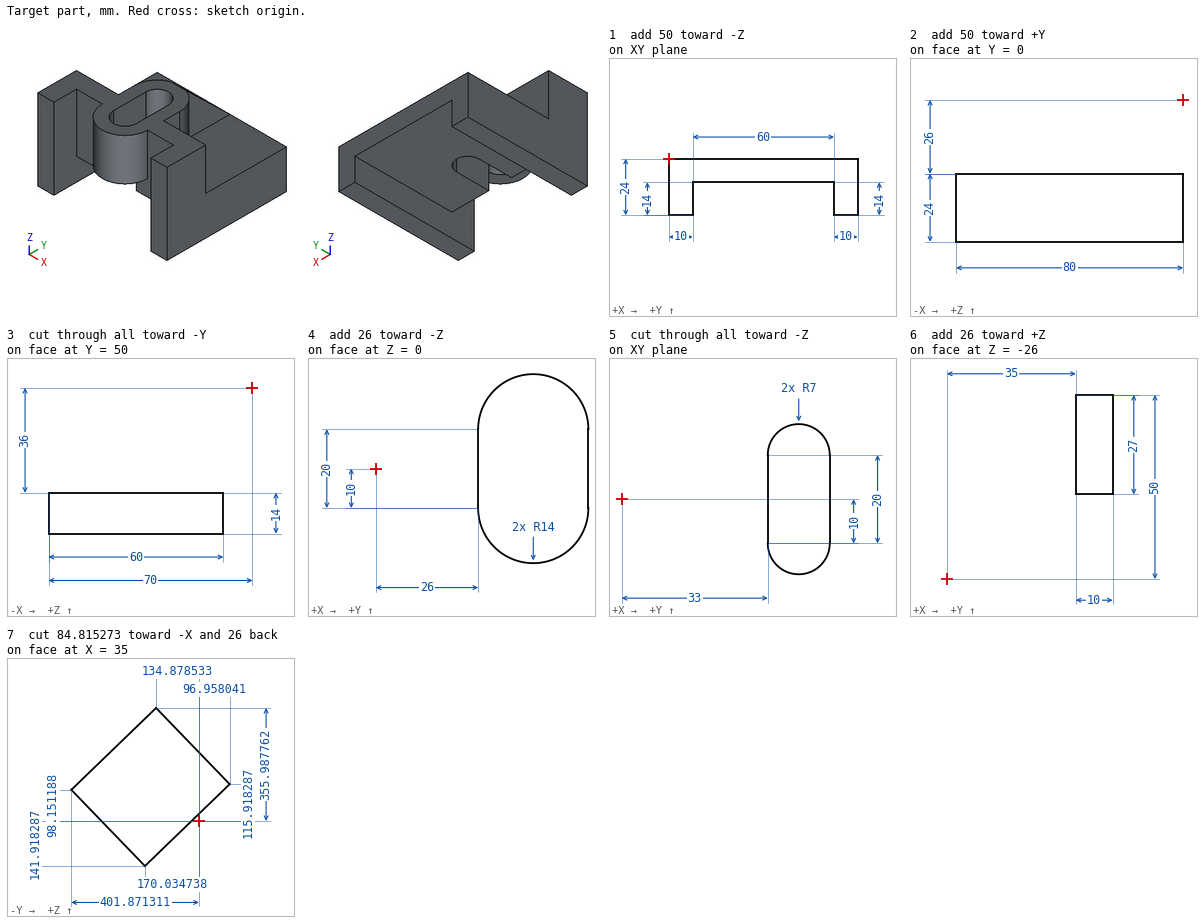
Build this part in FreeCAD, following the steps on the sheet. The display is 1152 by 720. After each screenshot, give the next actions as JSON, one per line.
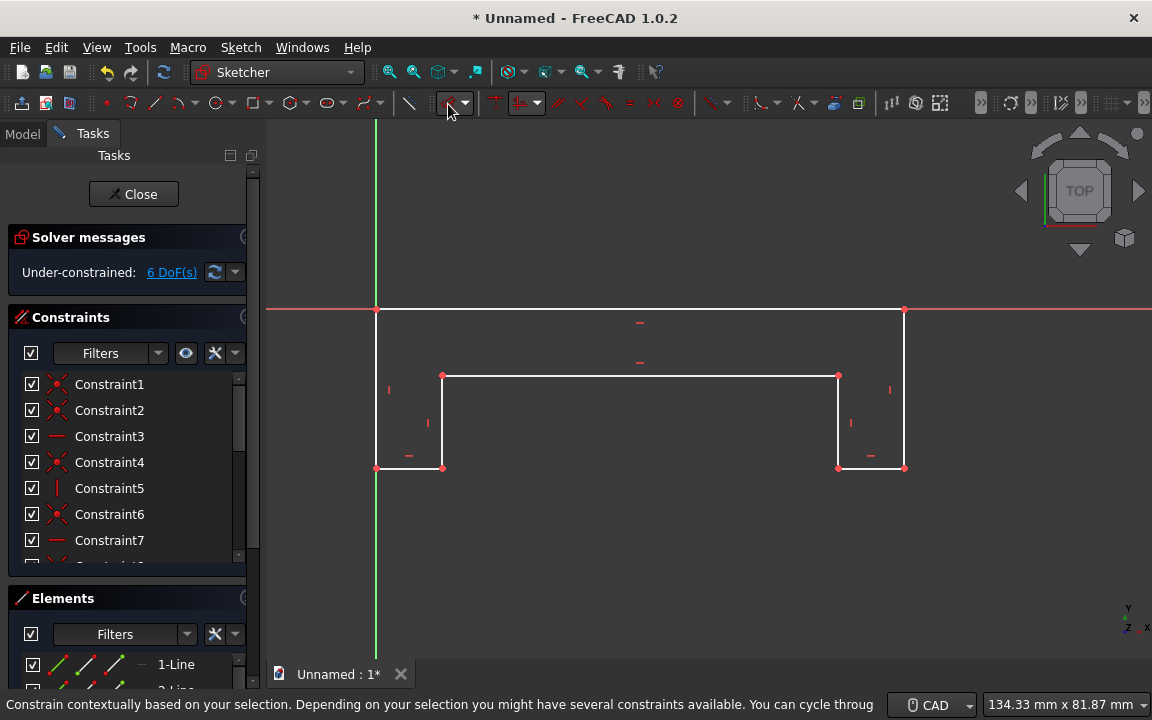
{"action": "left_click", "coordinate": [376, 357]}
{"action": "left_click", "coordinate": [342, 389]}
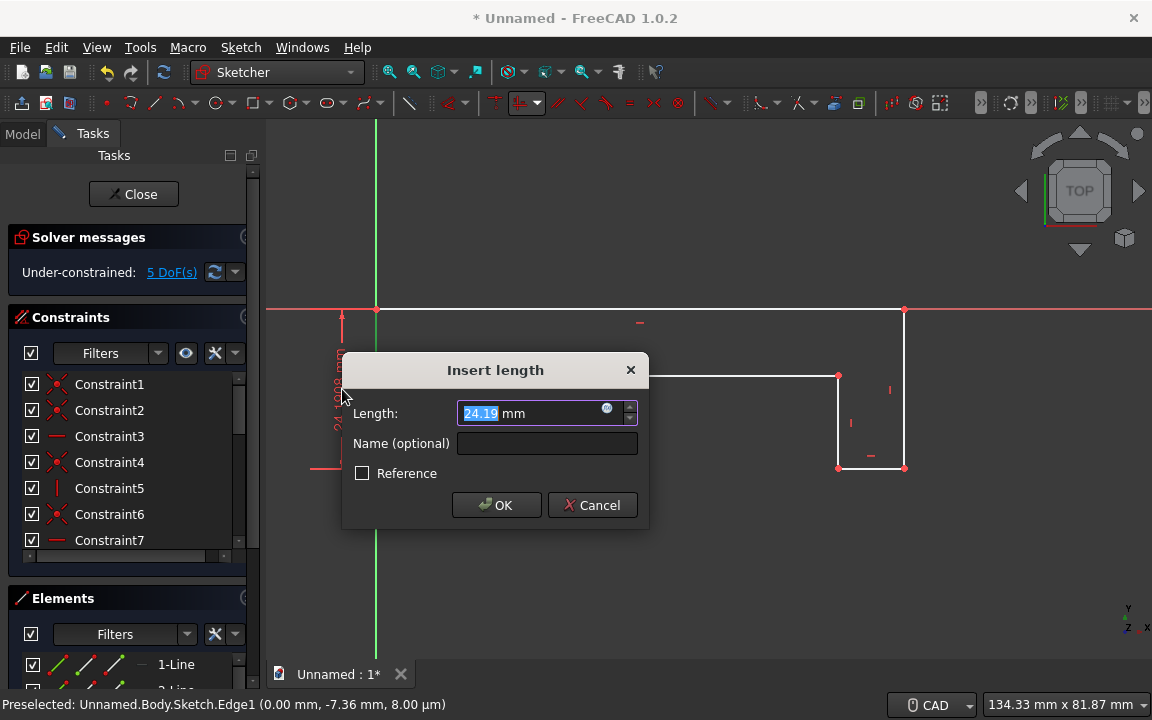
{"action": "type", "text": "24"}
{"action": "key", "text": "Return"}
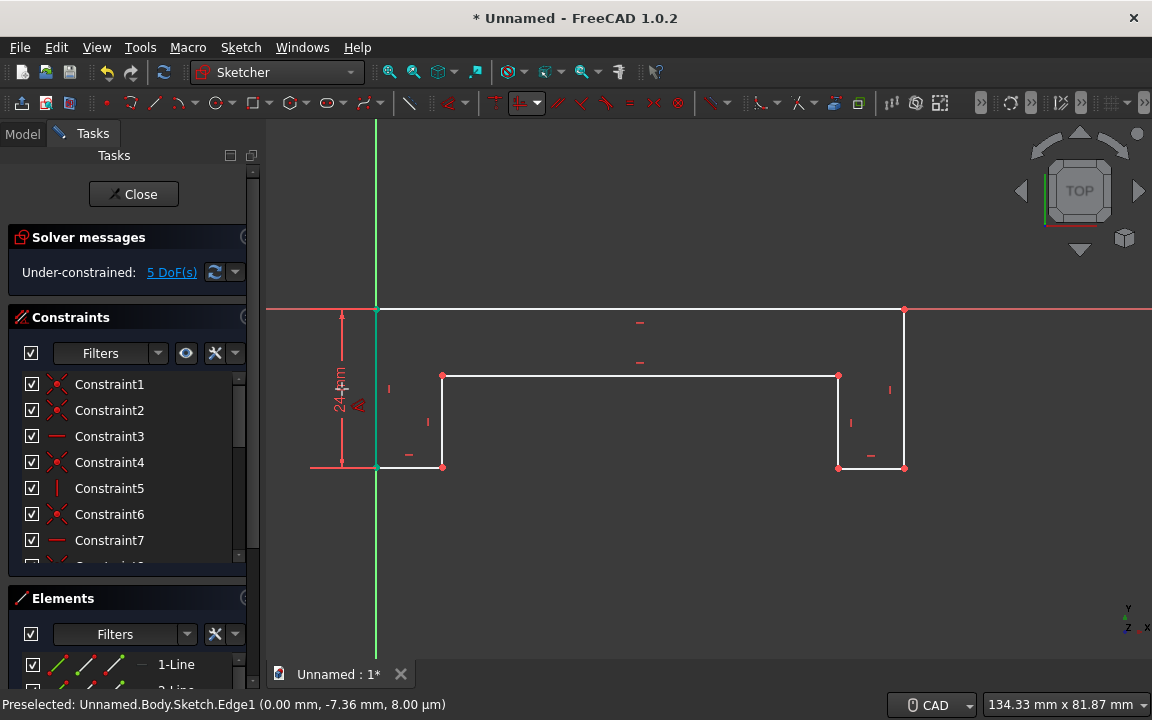
{"action": "left_click", "coordinate": [396, 468]}
{"action": "left_click", "coordinate": [409, 502]}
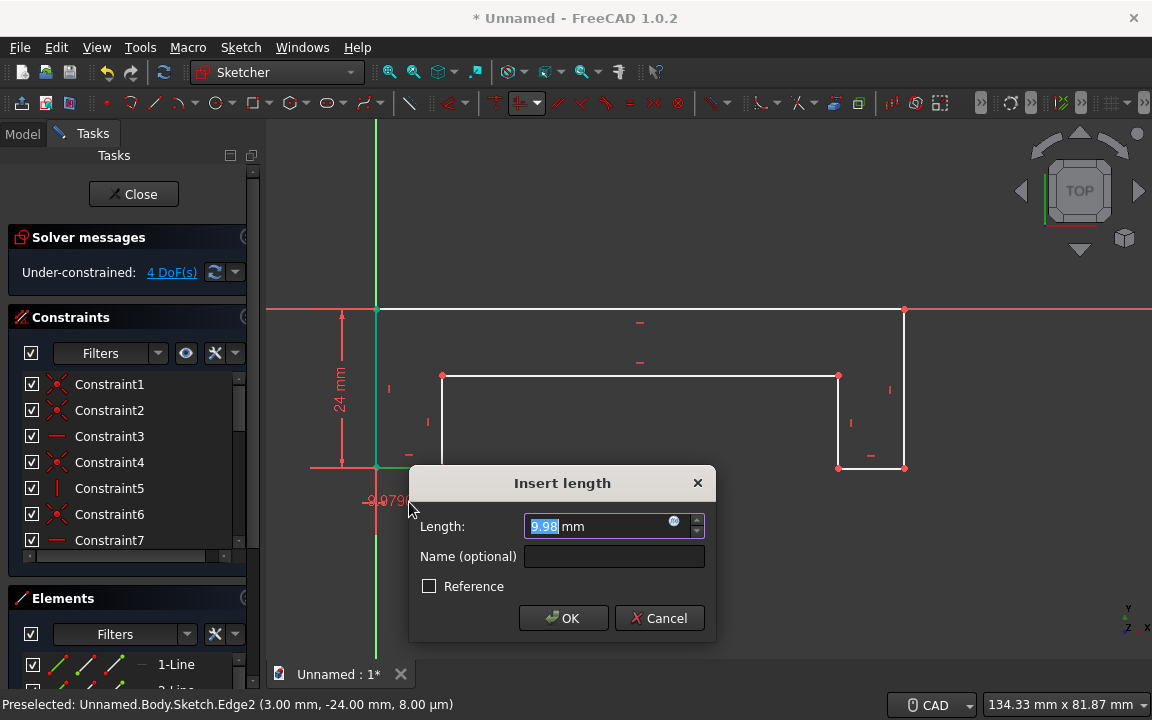
{"action": "type", "text": "10"}
{"action": "key", "text": "Return"}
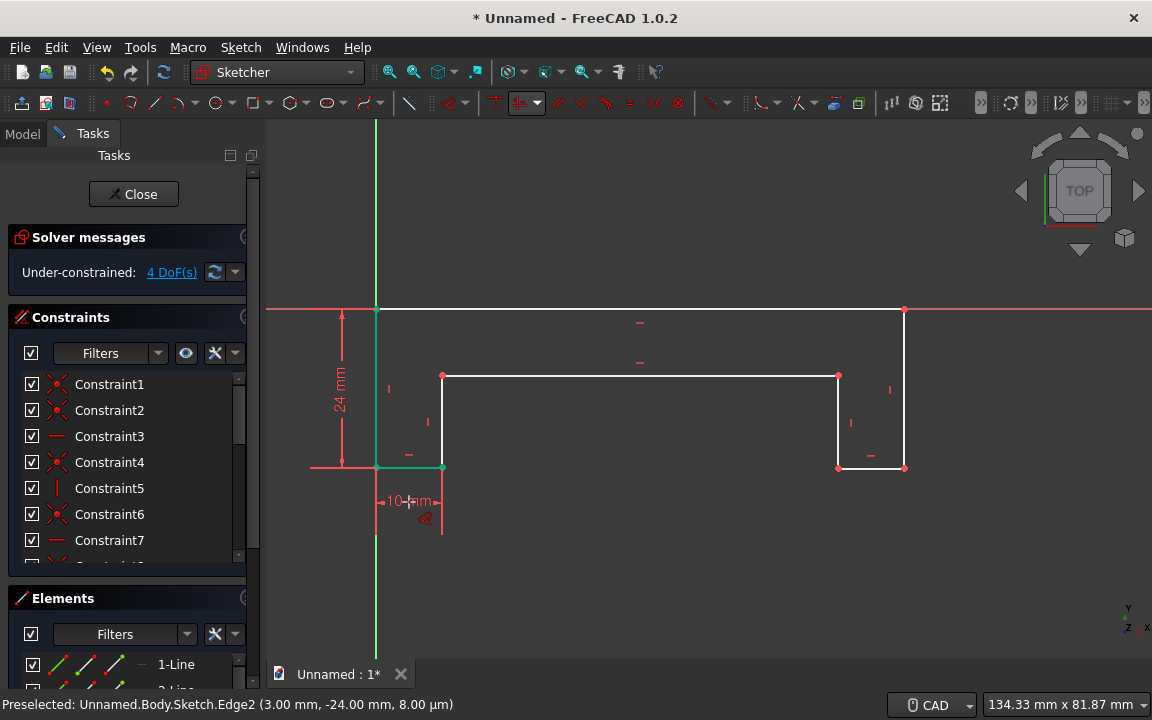
{"action": "left_click", "coordinate": [442, 440]}
{"action": "left_click", "coordinate": [408, 422]}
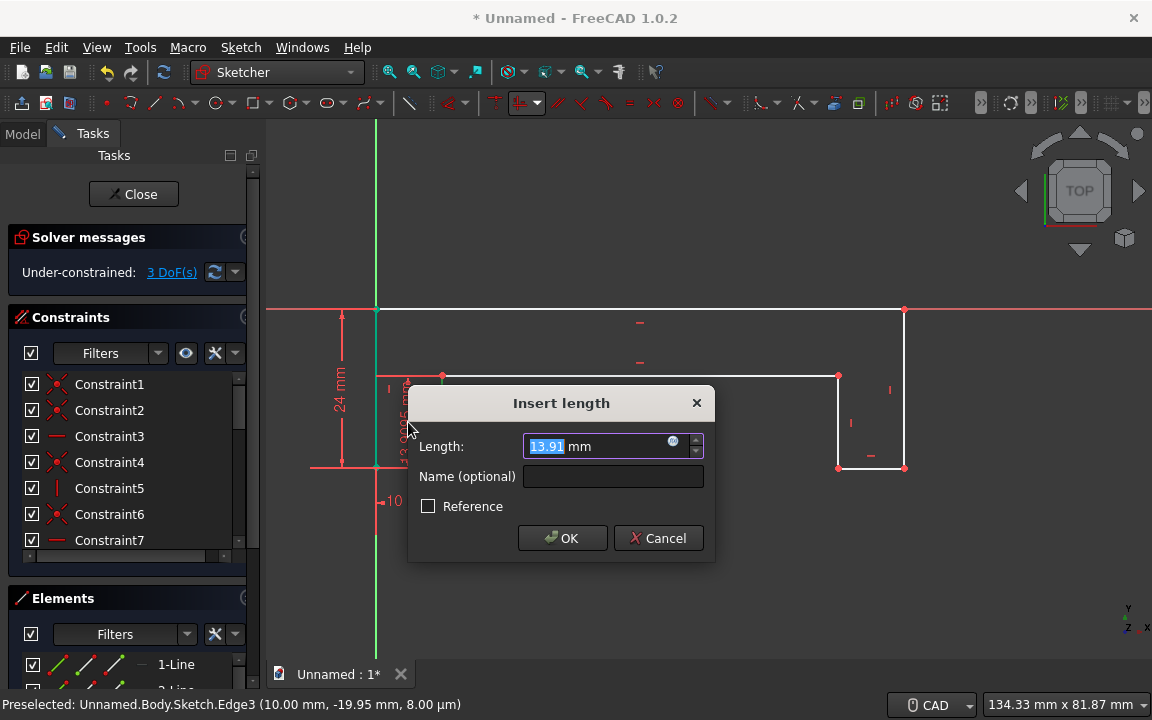
{"action": "type", "text": "14"}
{"action": "key", "text": "Return"}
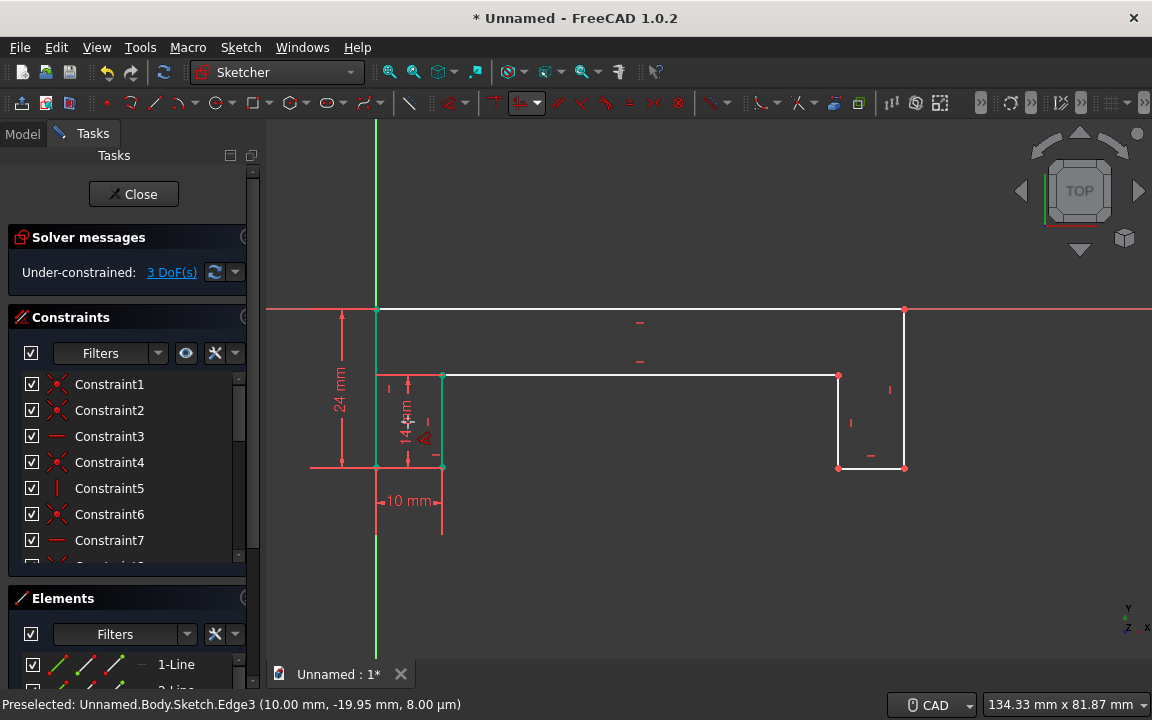
{"action": "left_click", "coordinate": [561, 375]}
{"action": "left_click", "coordinate": [640, 341]}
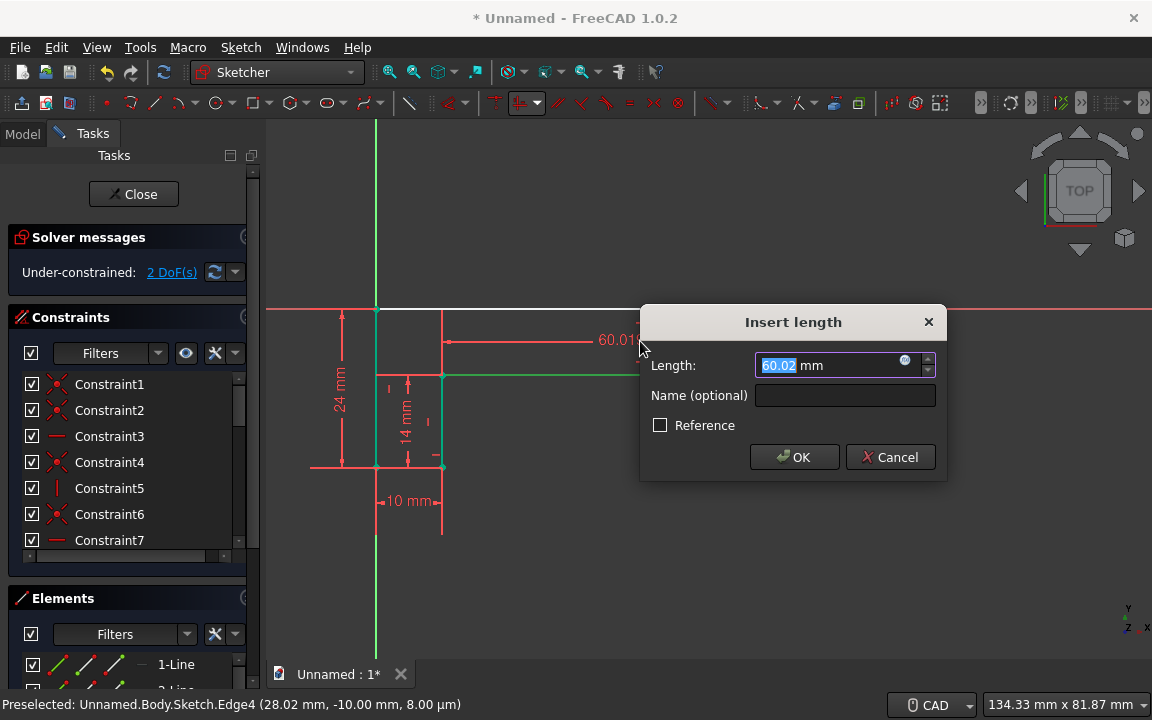
{"action": "type", "text": "60"}
{"action": "key", "text": "Return"}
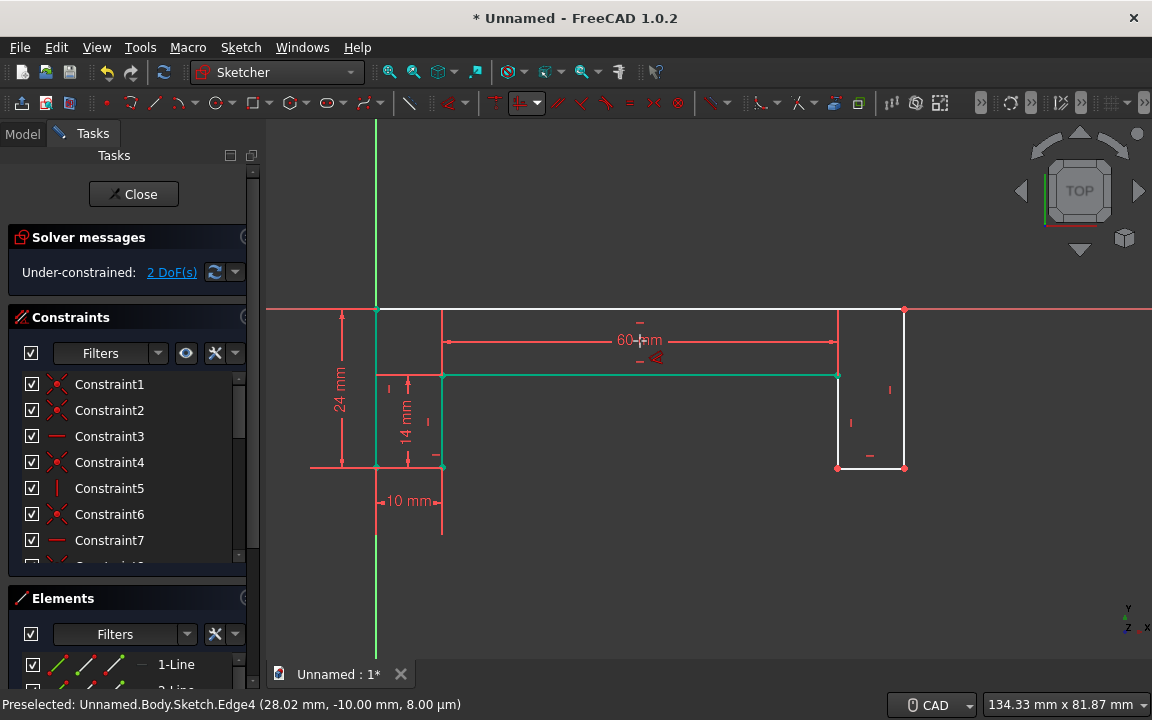
{"action": "left_click", "coordinate": [838, 403]}
{"action": "left_click", "coordinate": [872, 422]}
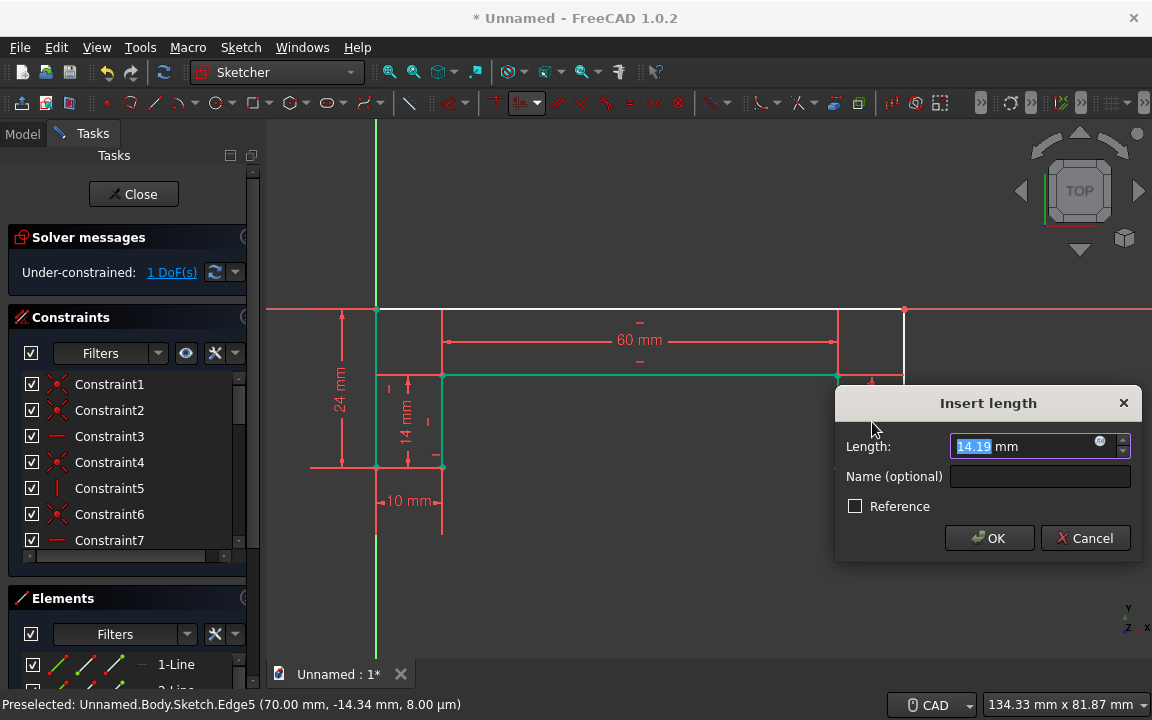
{"action": "type", "text": "14"}
{"action": "key", "text": "Return"}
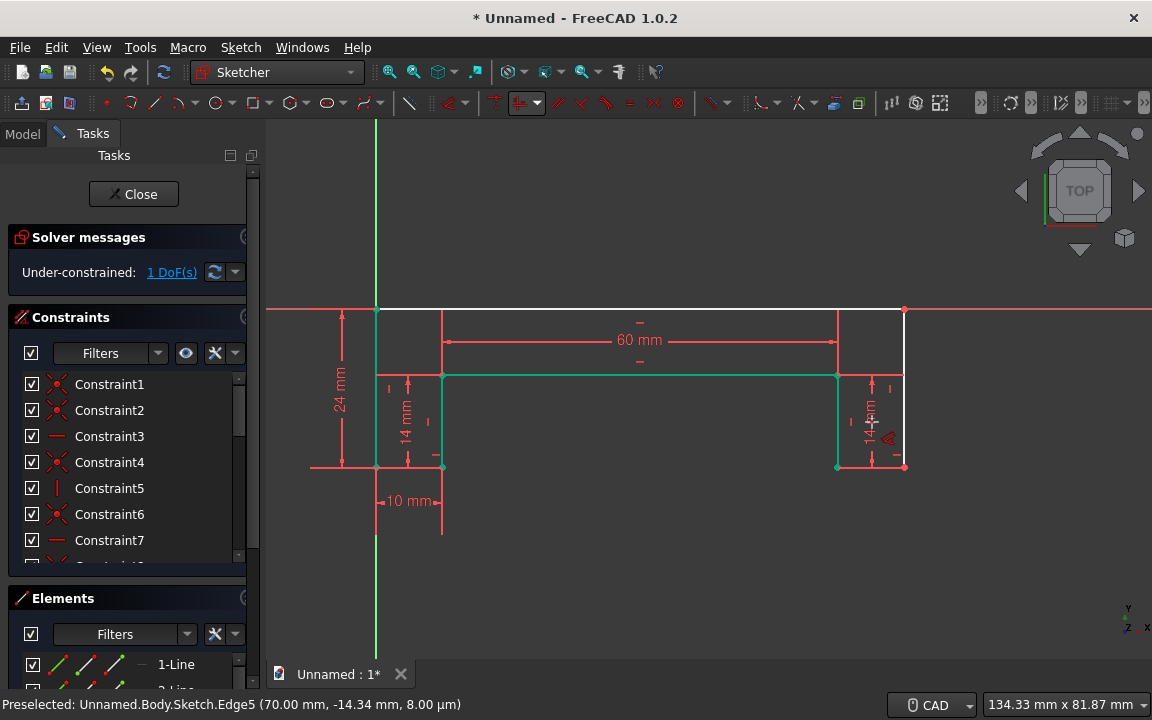
{"action": "left_click", "coordinate": [858, 468]}
{"action": "left_click", "coordinate": [871, 502]}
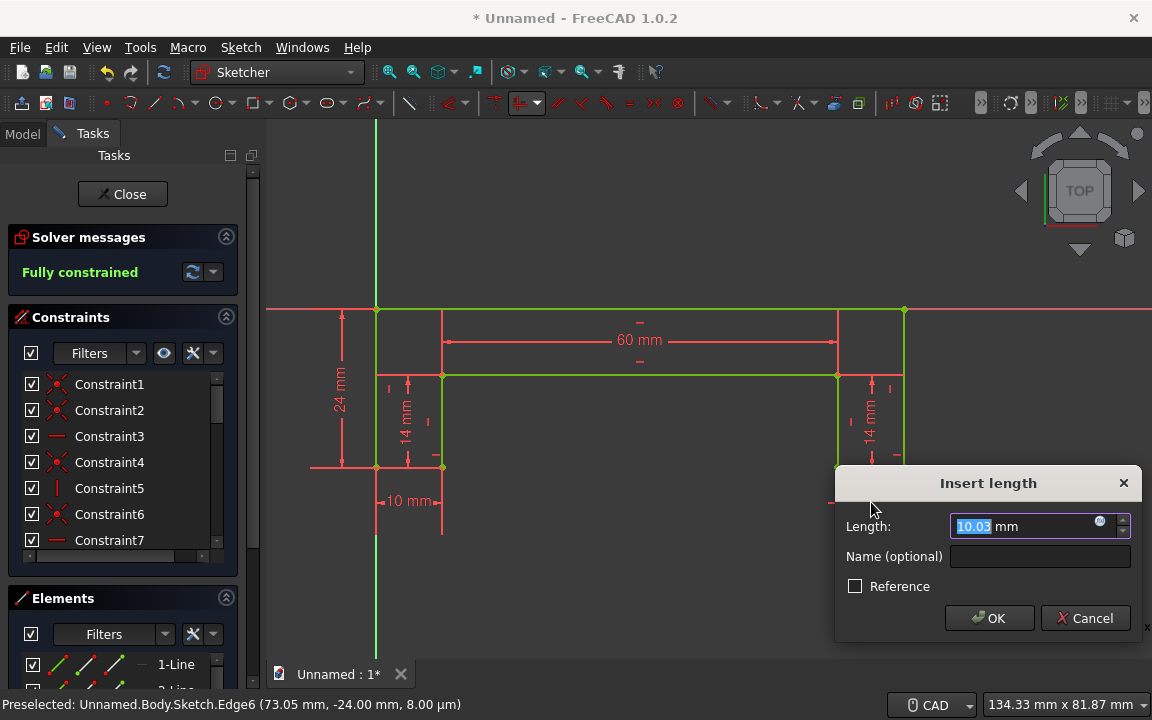
{"action": "type", "text": "10"}
{"action": "key", "text": "Return"}
{"action": "key", "text": "Escape"}